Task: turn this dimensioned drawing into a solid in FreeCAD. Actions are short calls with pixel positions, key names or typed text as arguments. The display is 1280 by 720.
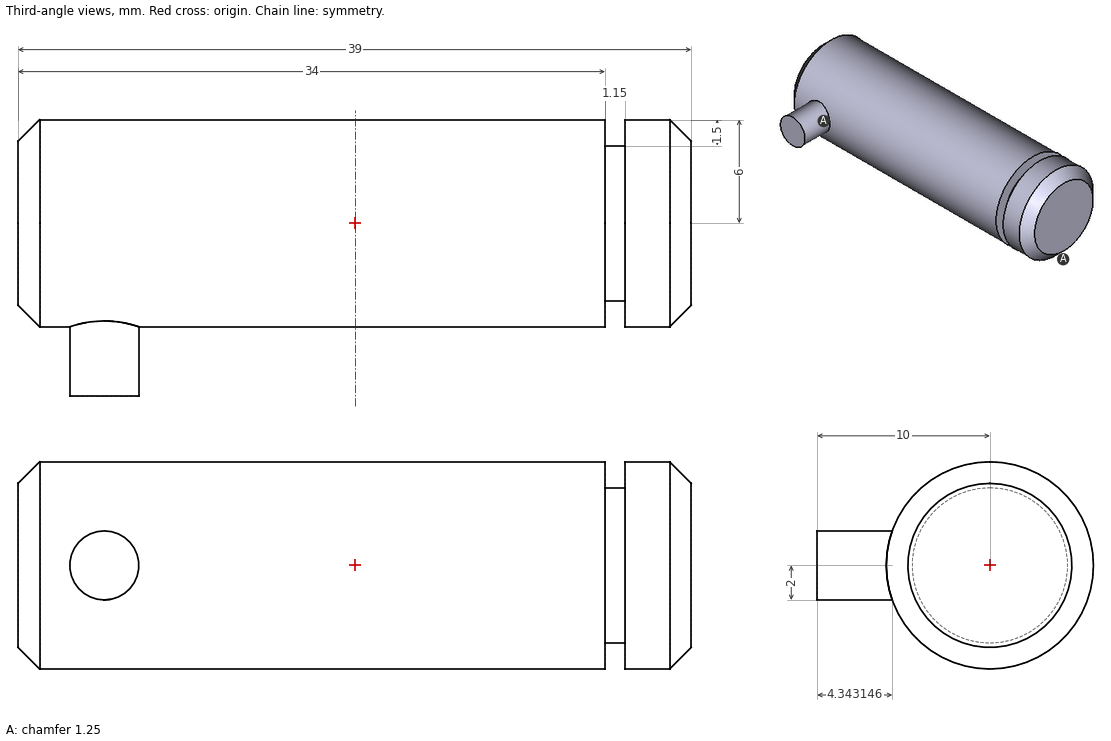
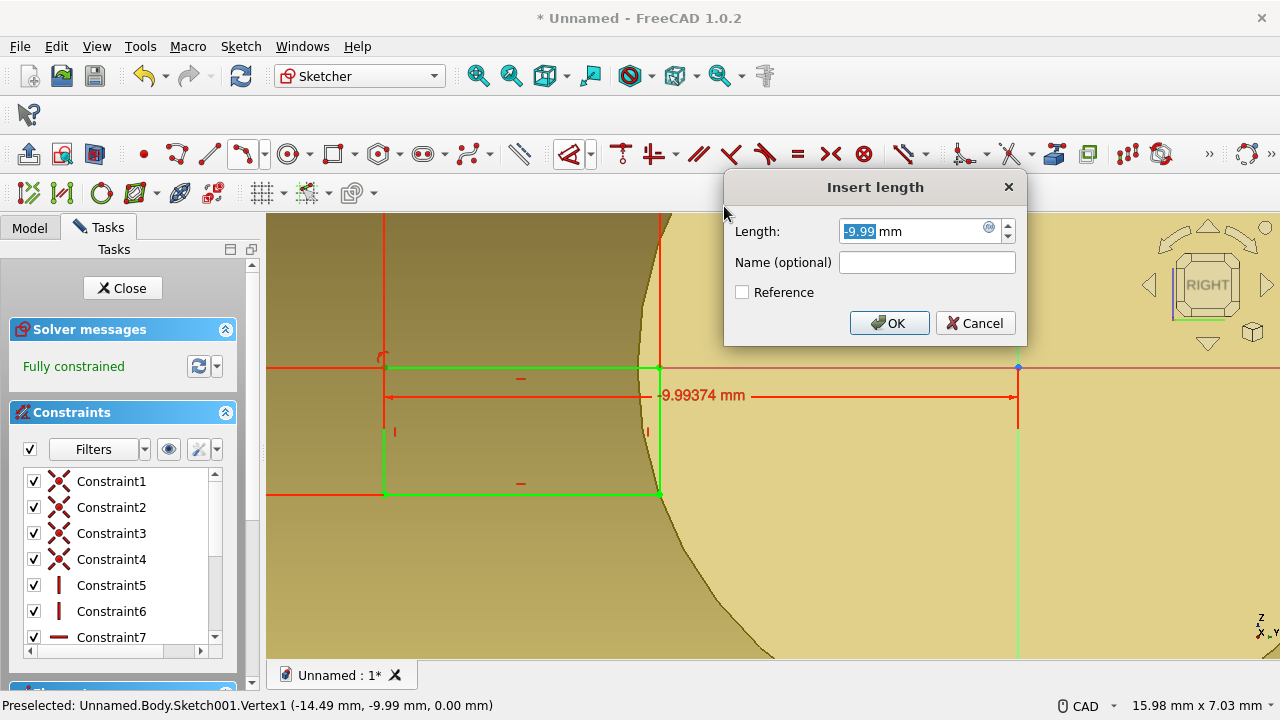
text(-10)
key(Return)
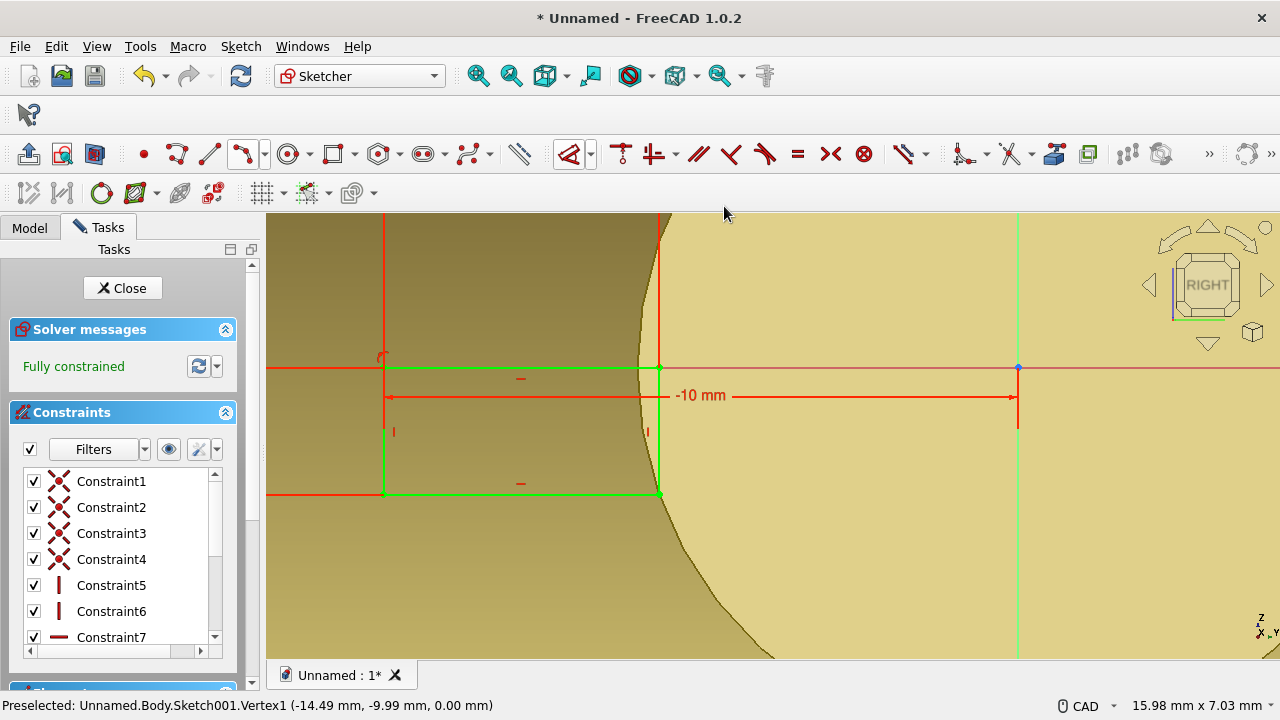
click(123, 288)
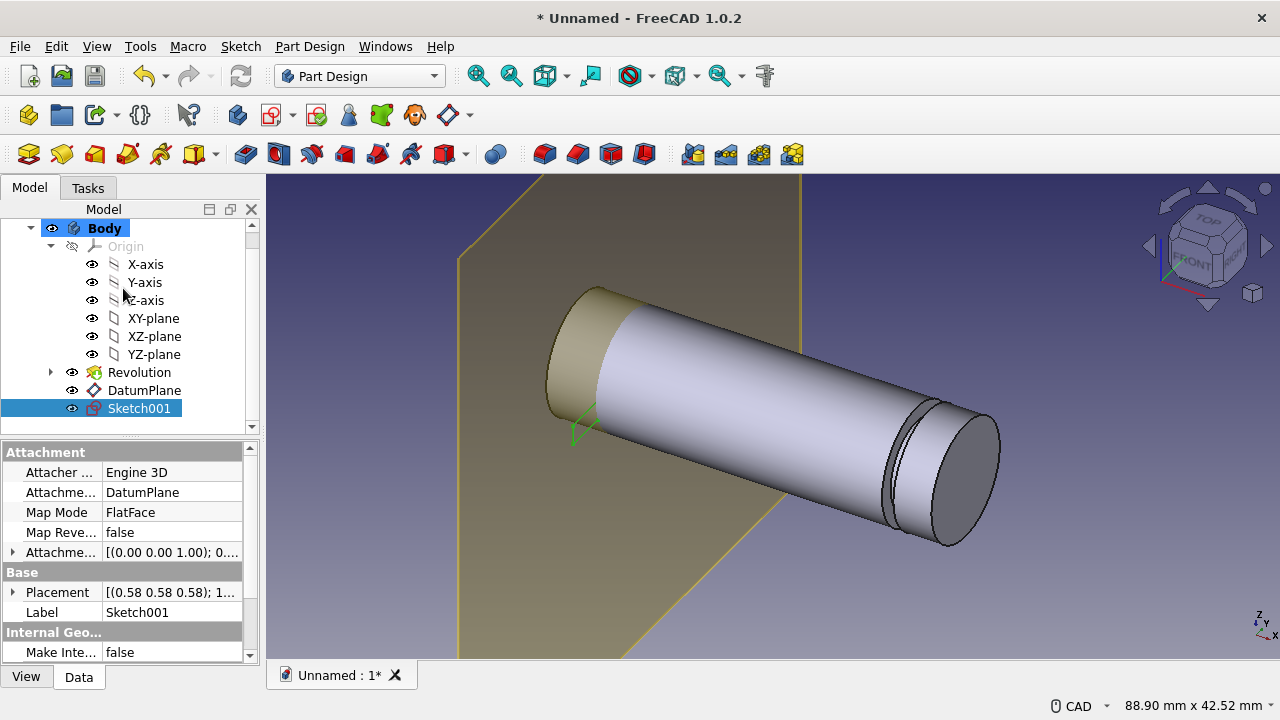
click(62, 154)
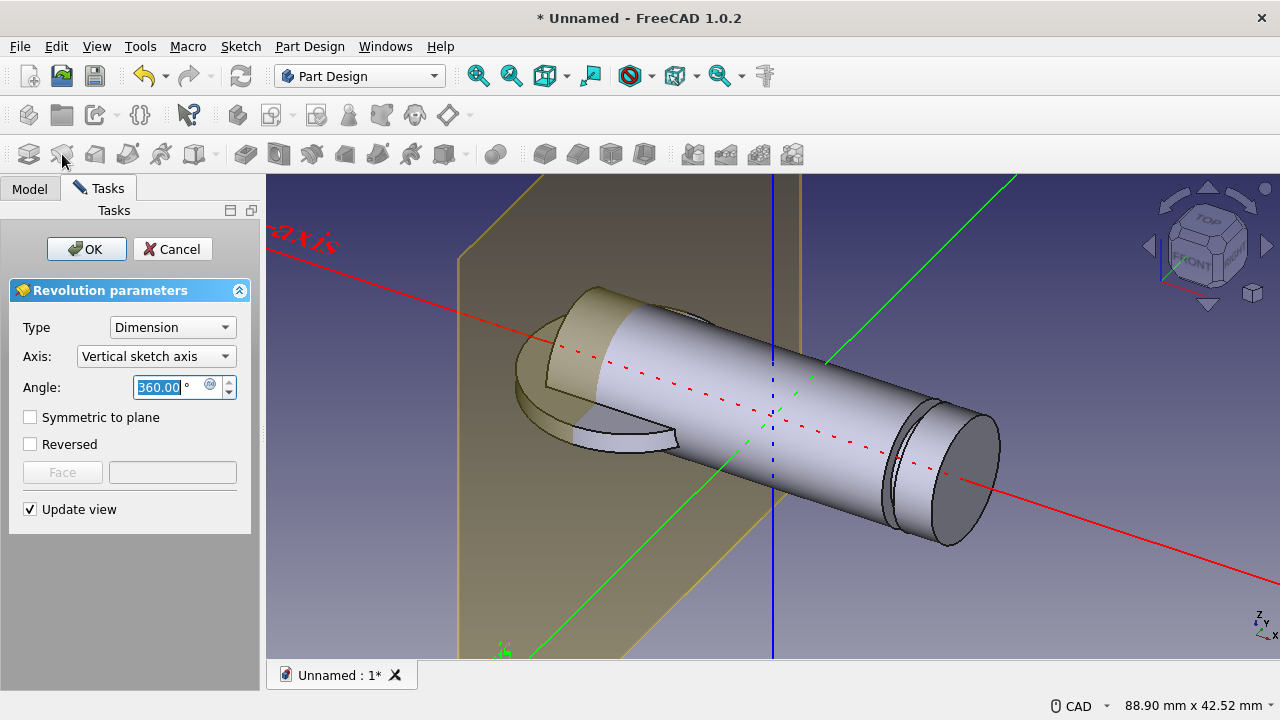
click(157, 356)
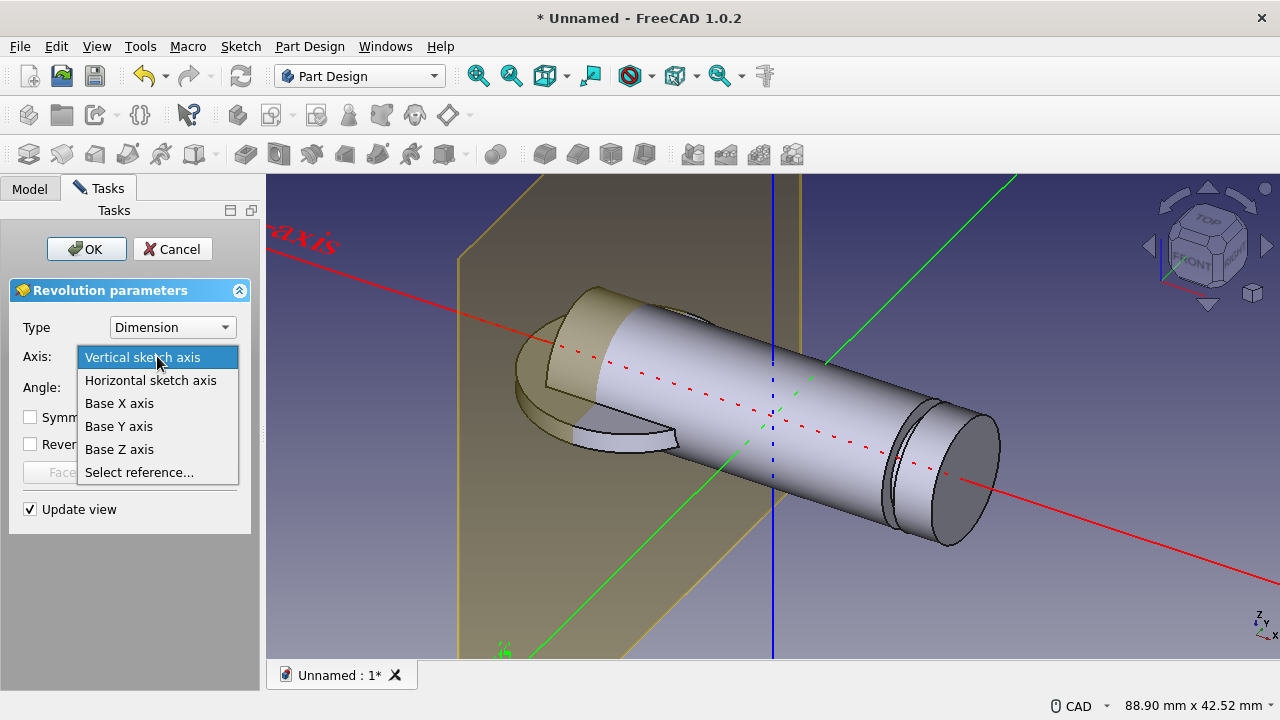
click(156, 380)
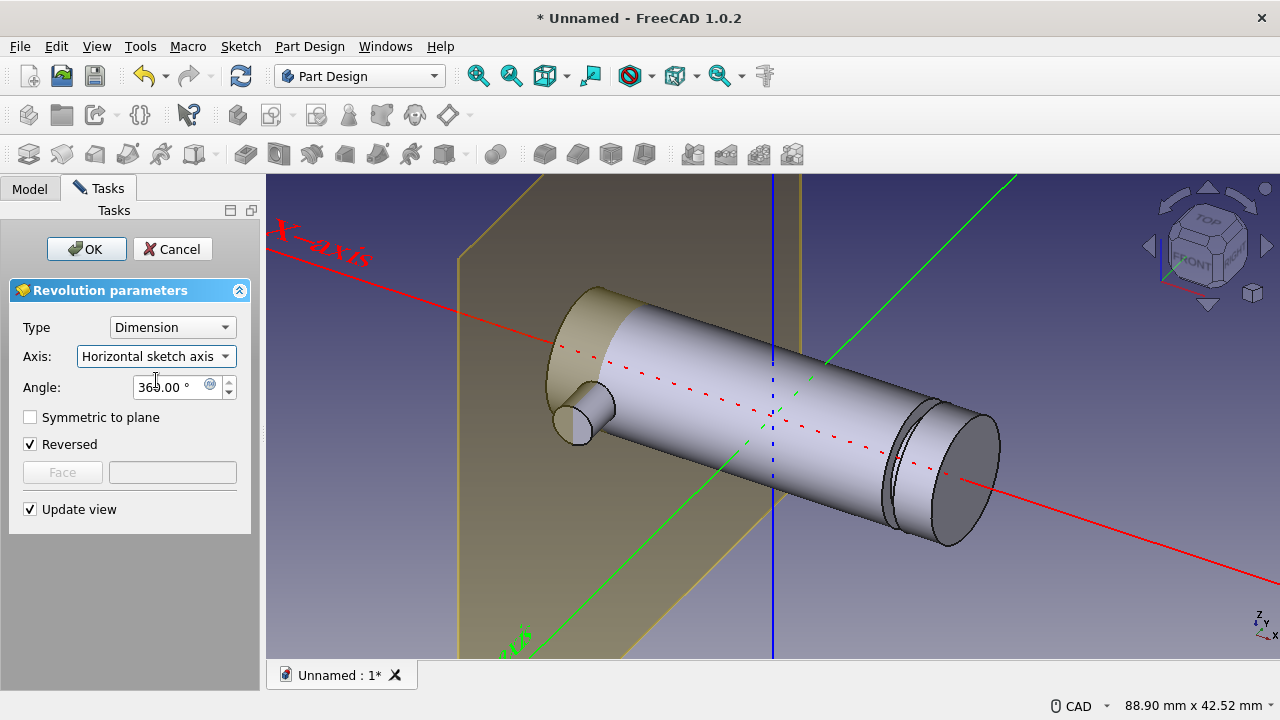
click(87, 249)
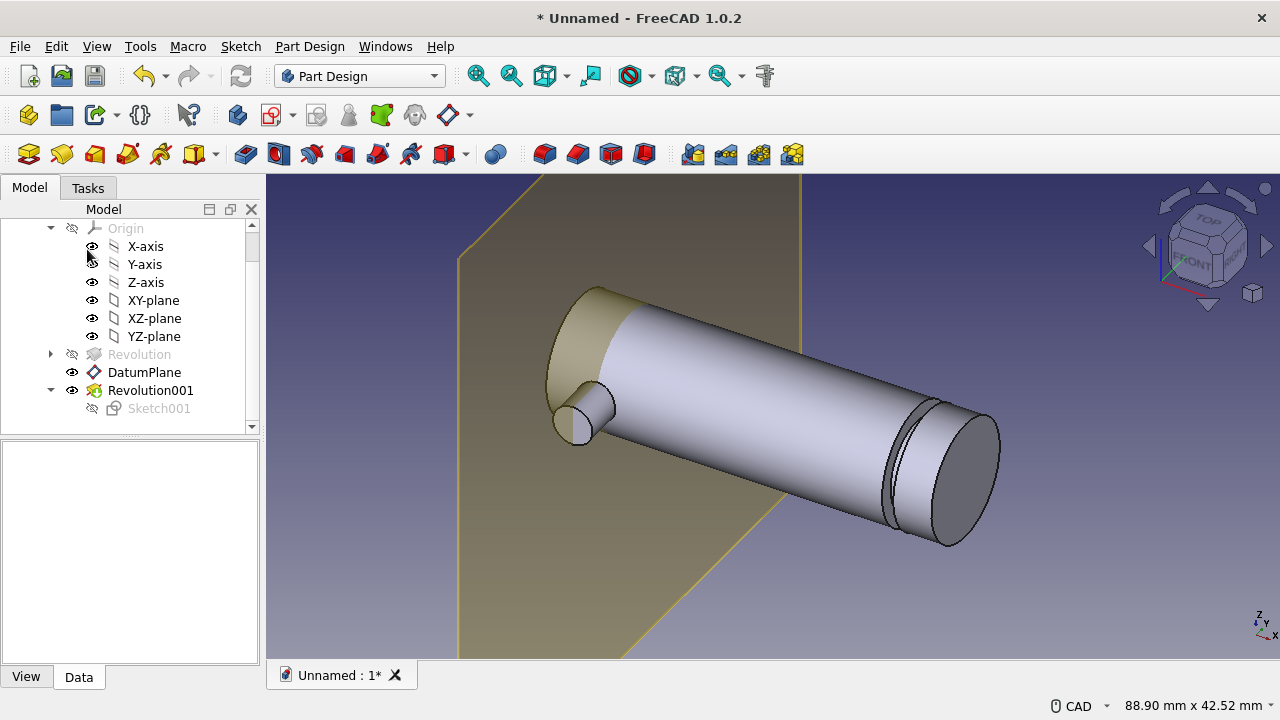
click(117, 372)
key(space)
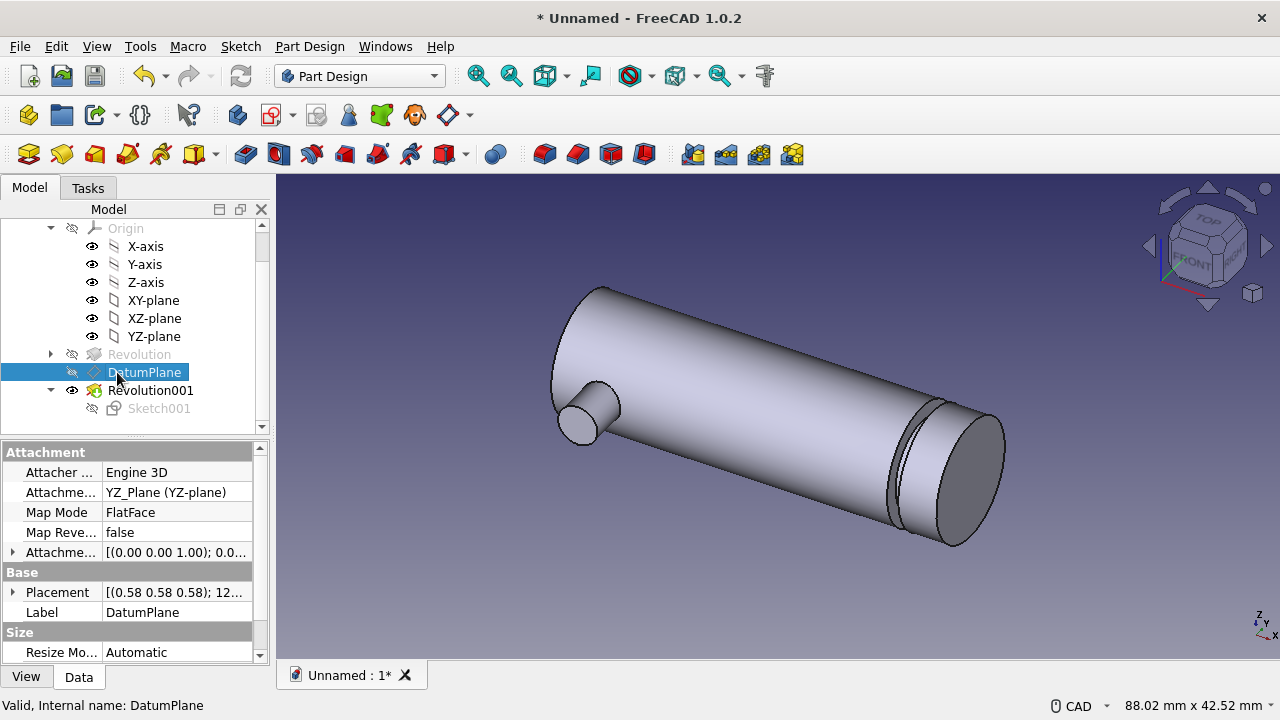
click(936, 513)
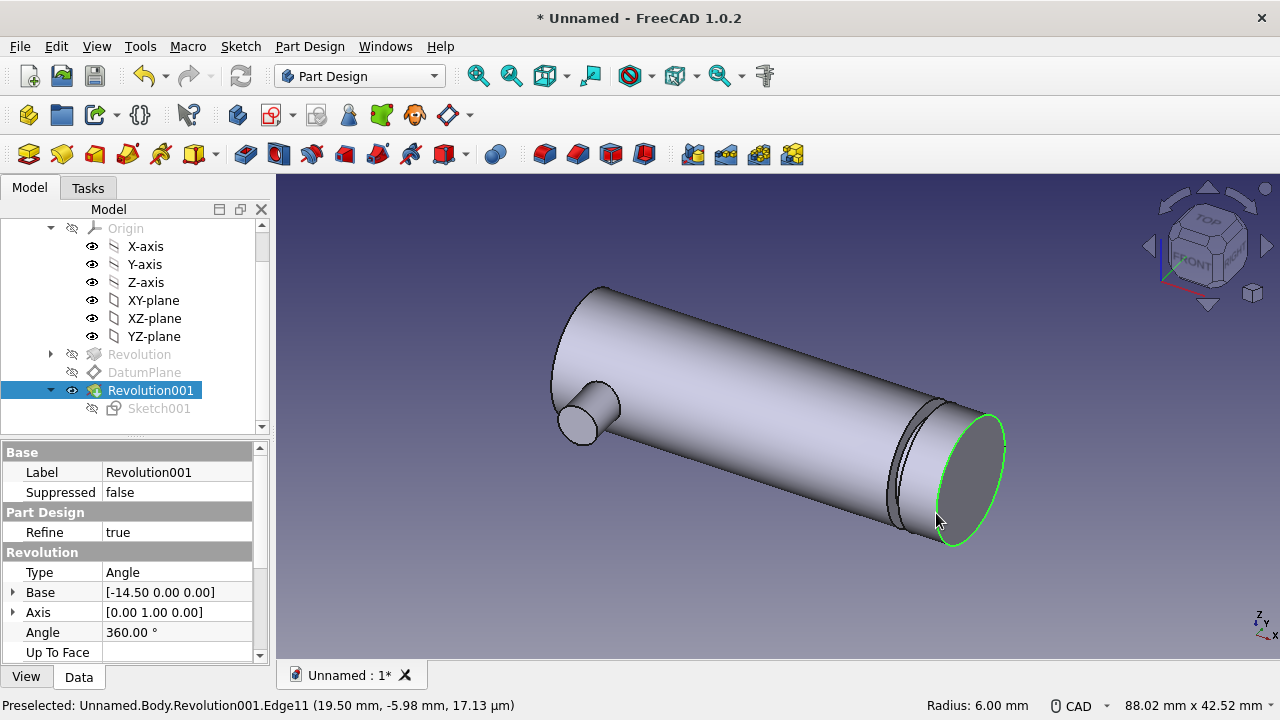
click(596, 288, ctrl)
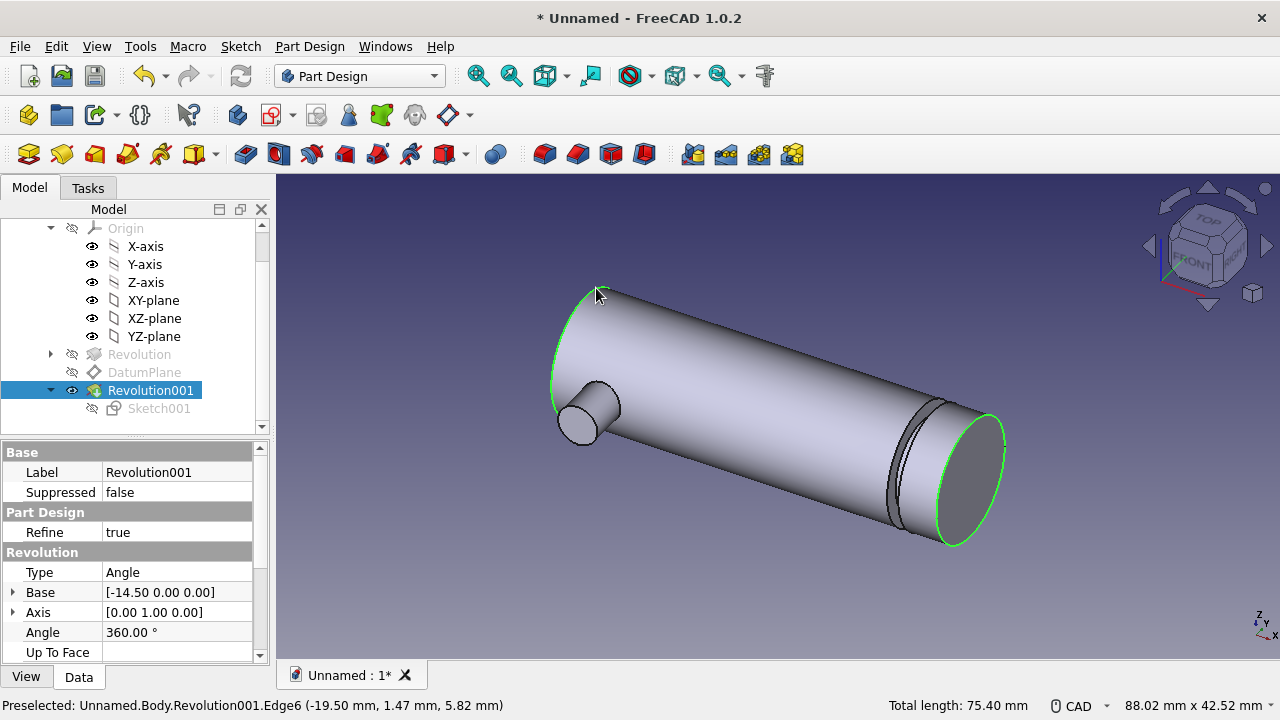
click(578, 154)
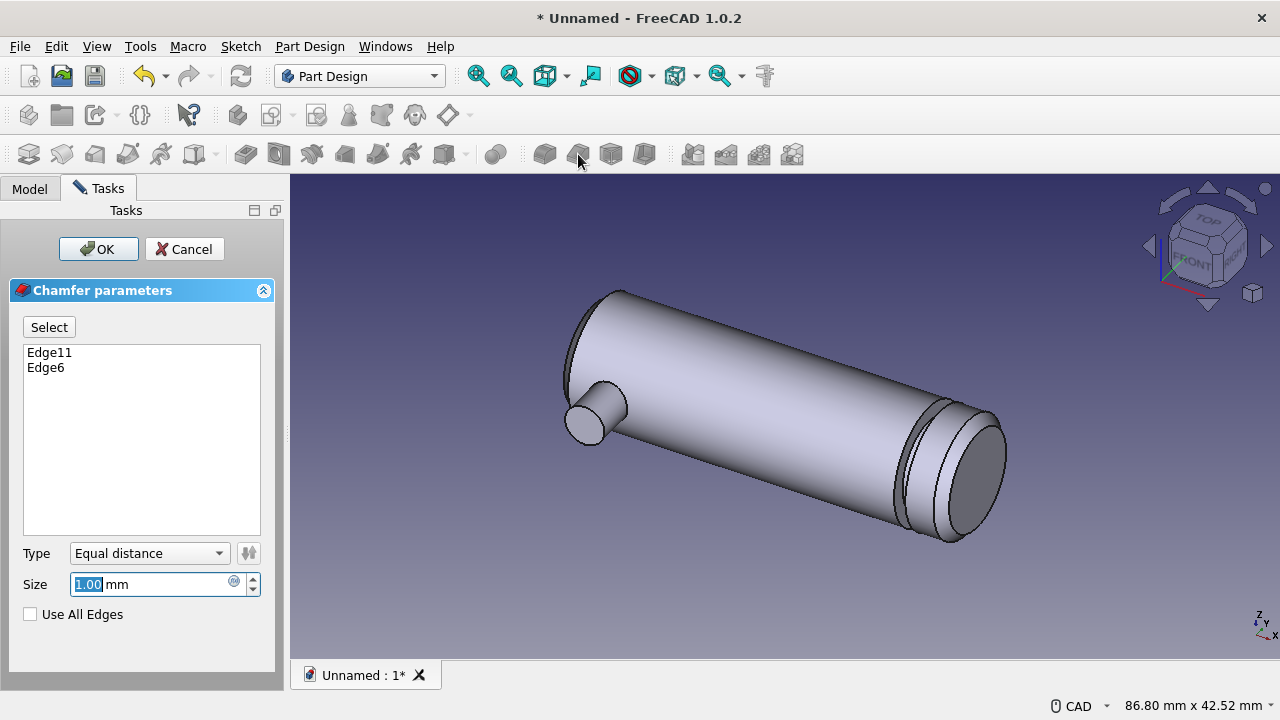
text(1.25)
key(Tab)